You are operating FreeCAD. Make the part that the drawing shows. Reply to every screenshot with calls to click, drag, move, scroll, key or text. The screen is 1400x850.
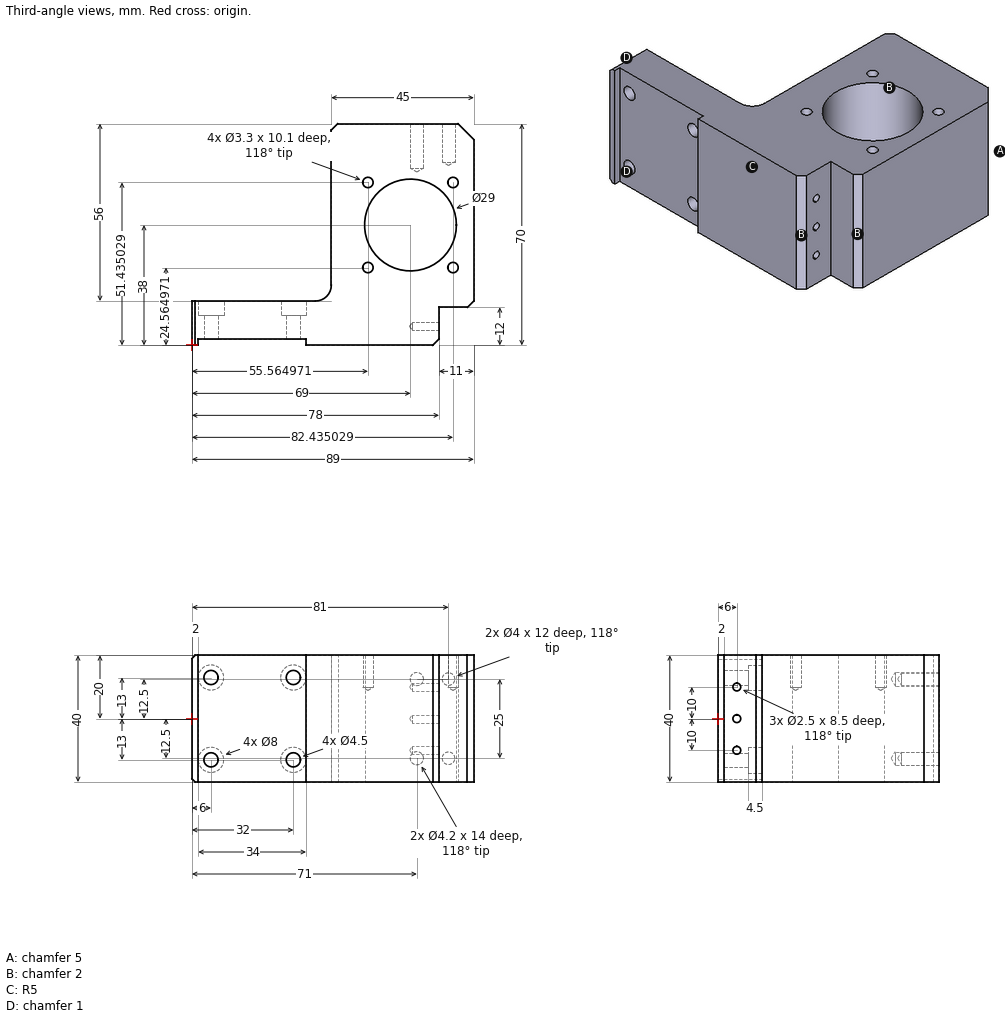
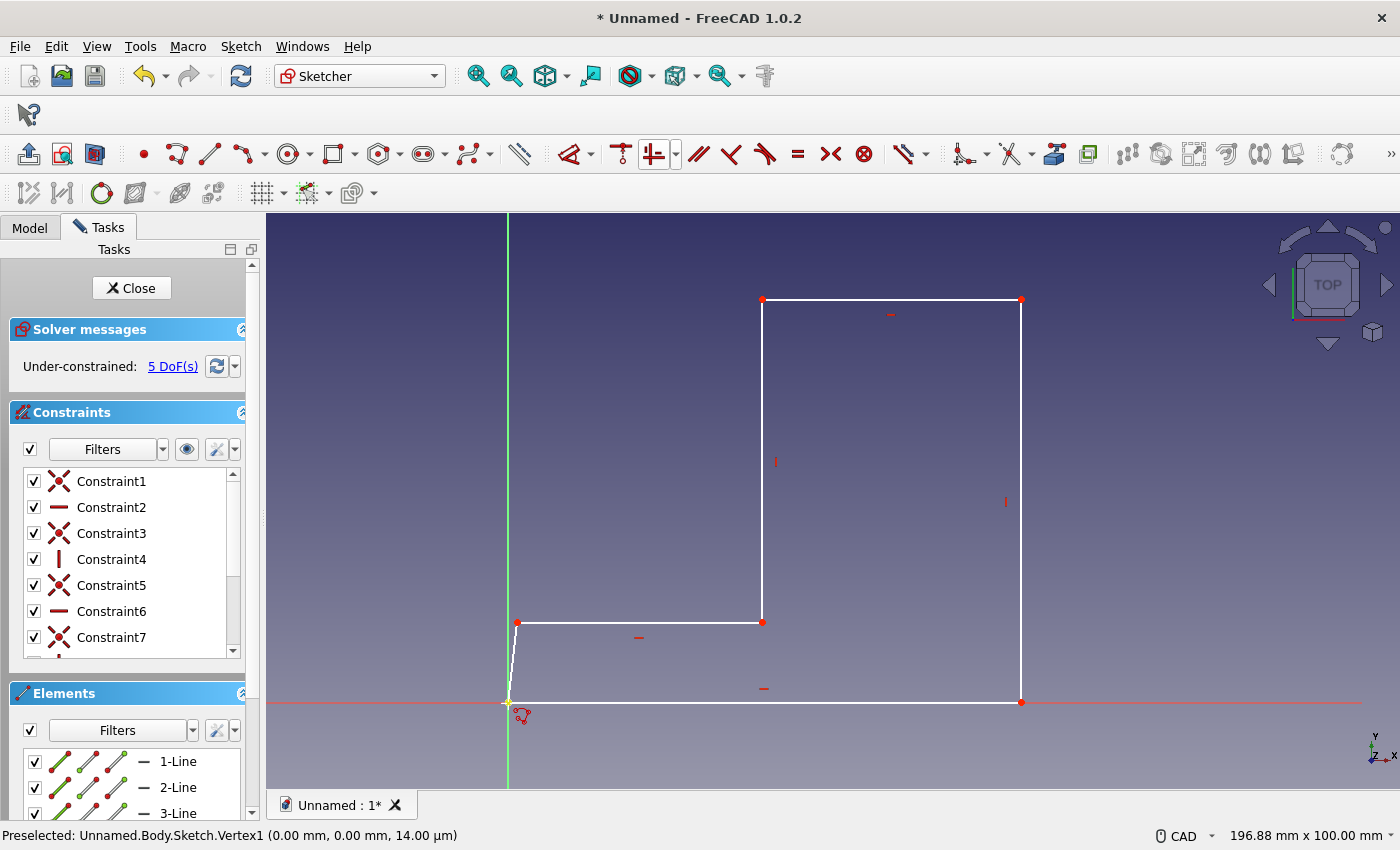
click(288, 154)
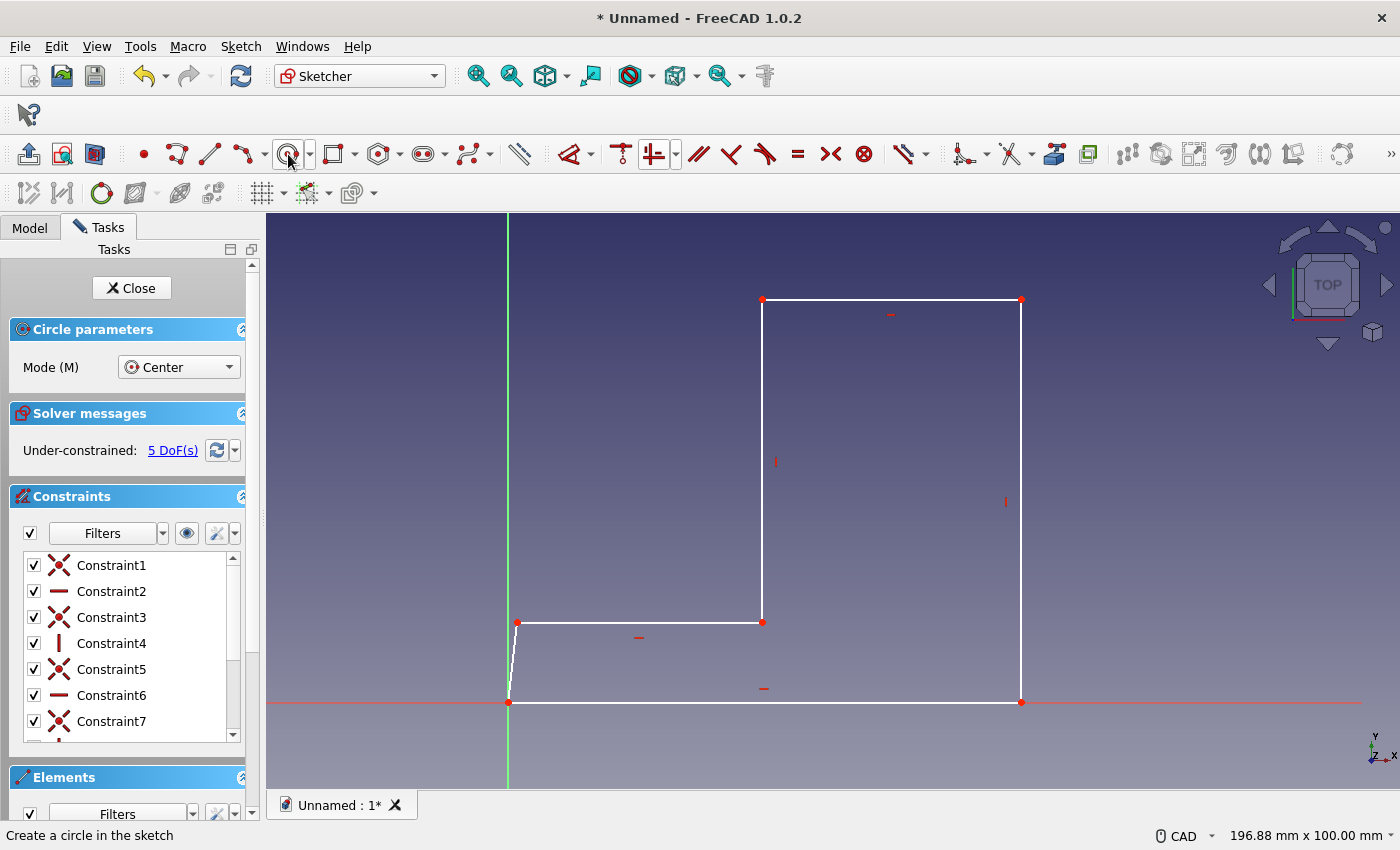
click(906, 484)
move(965, 425)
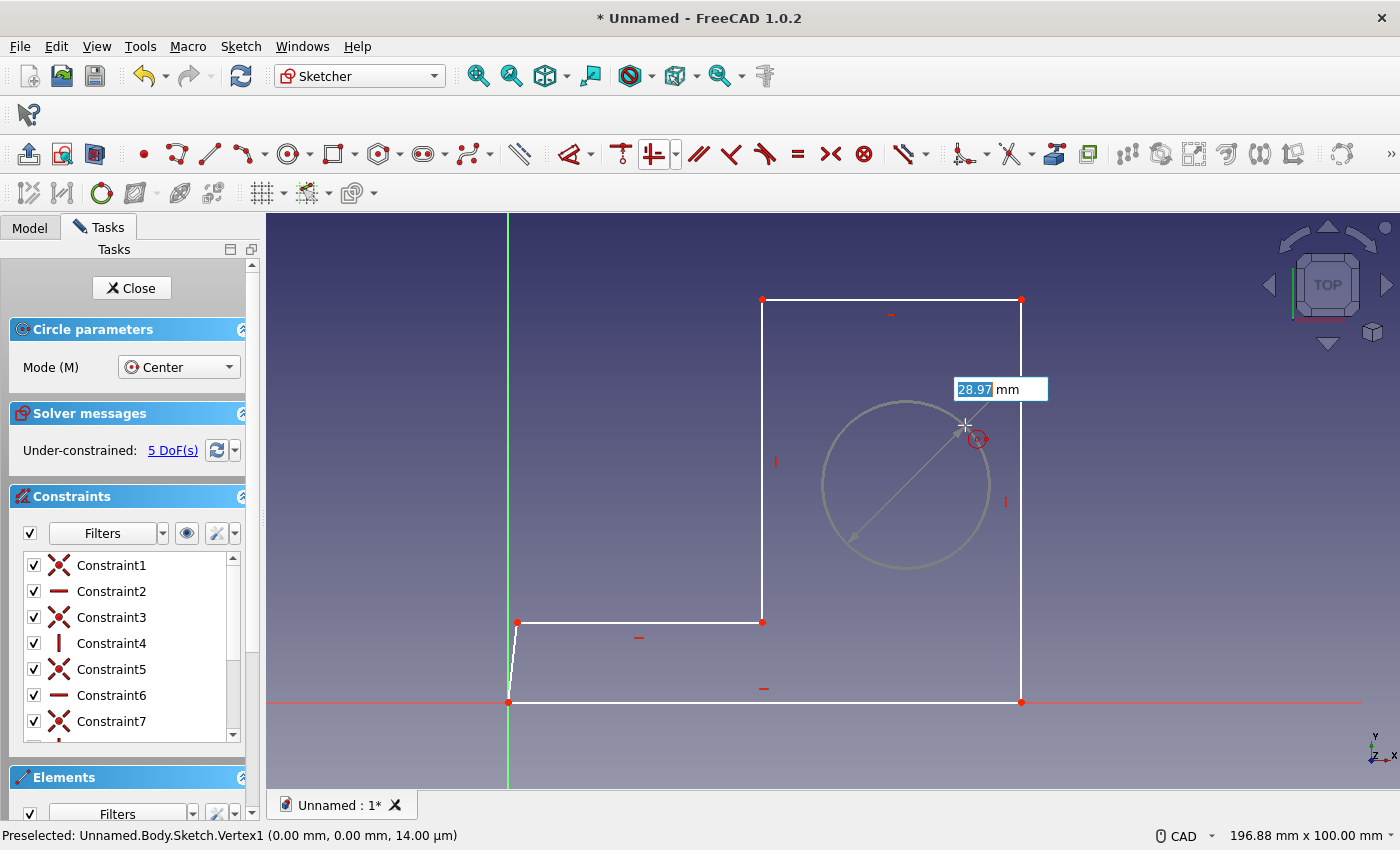
text(29)
key(Return)
key(Escape)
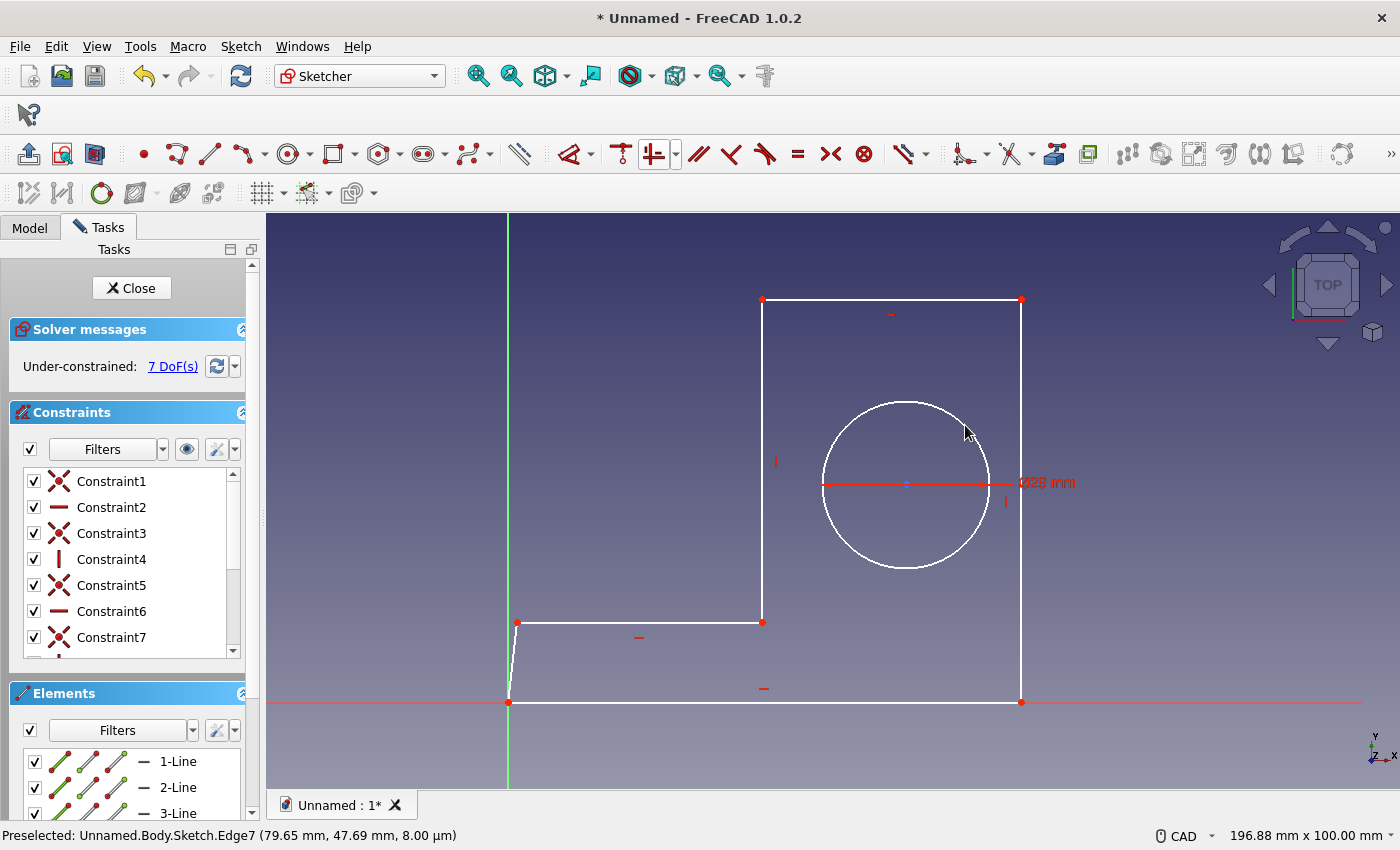
click(511, 679)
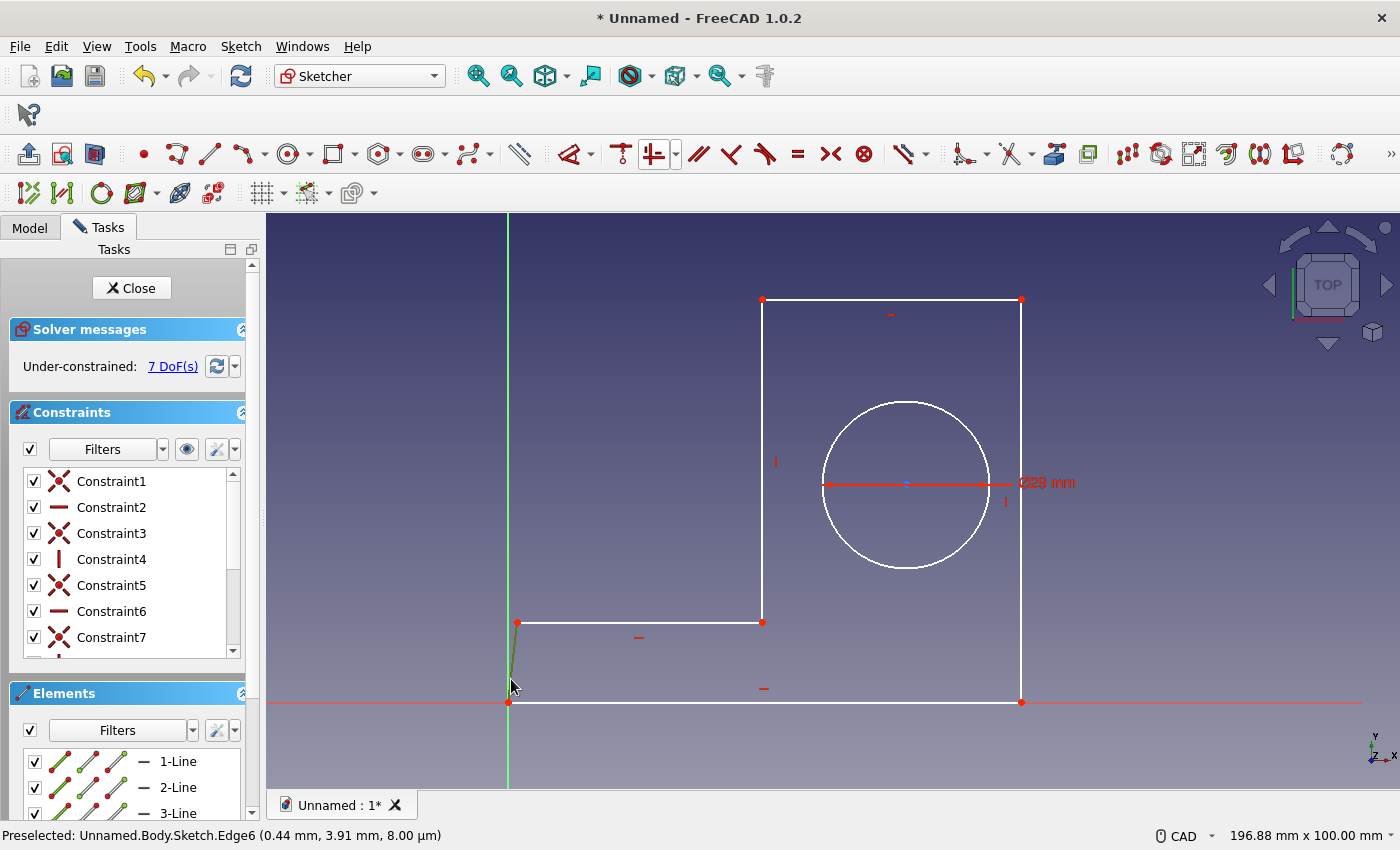
click(676, 154)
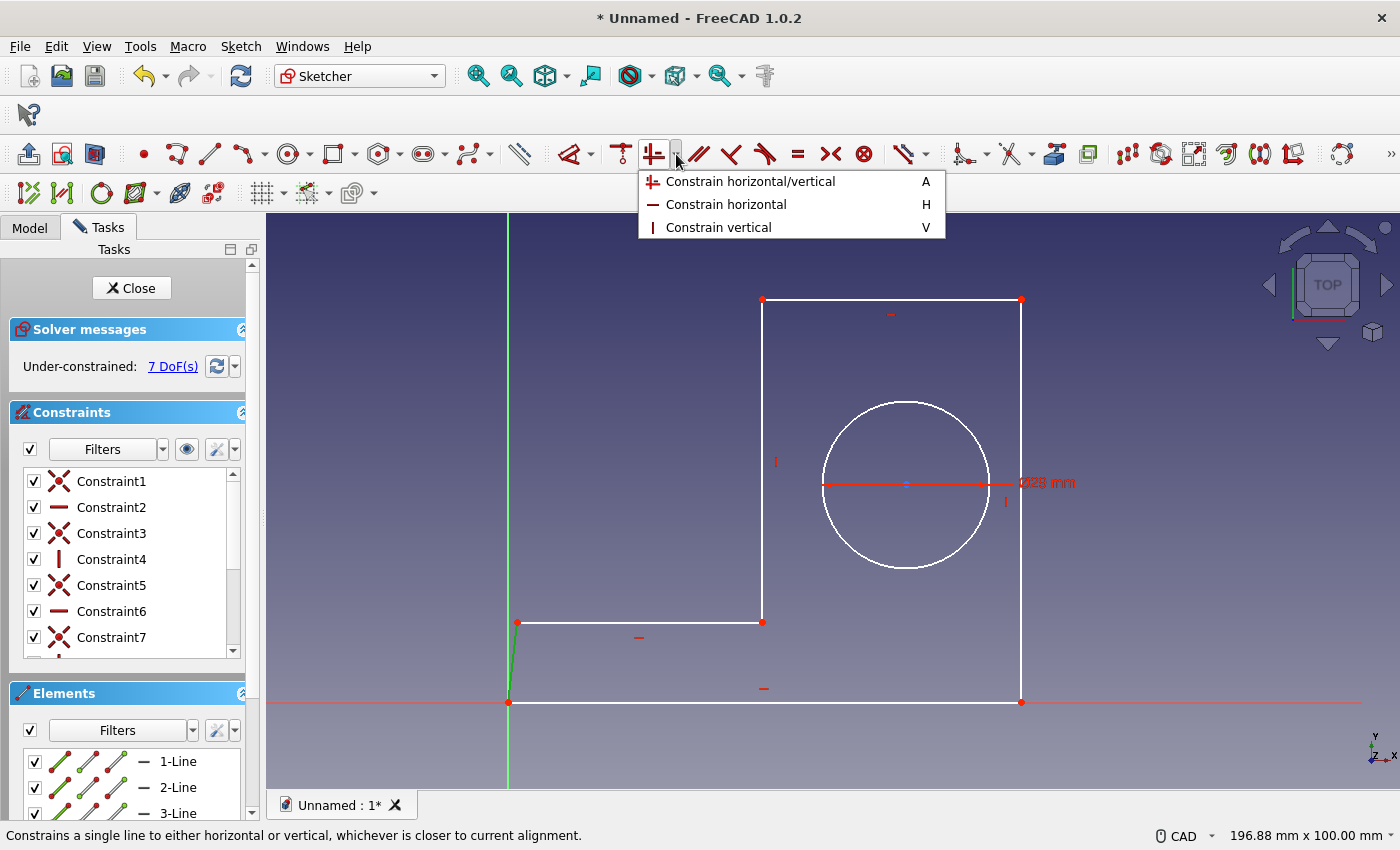
click(792, 228)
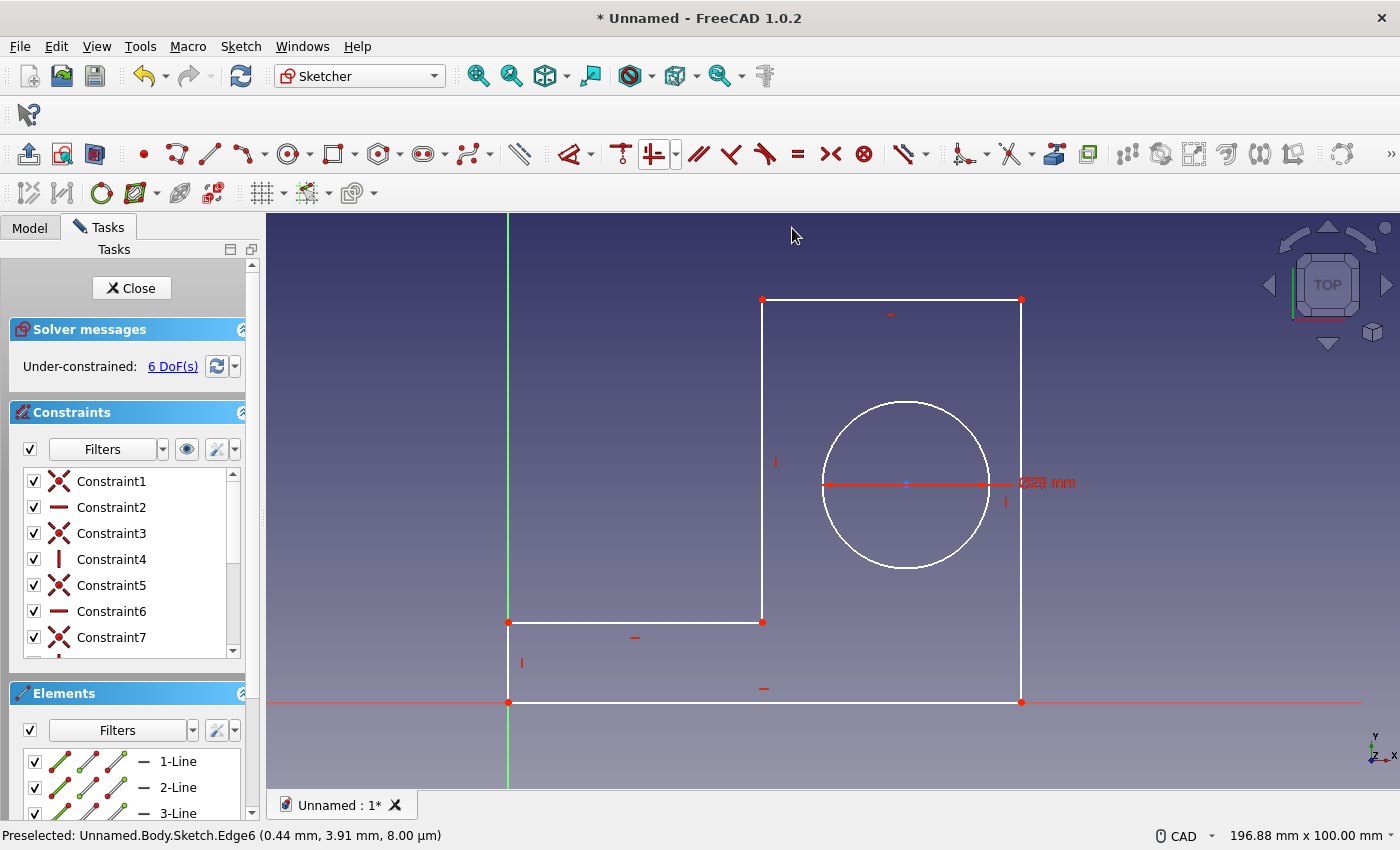
key(d)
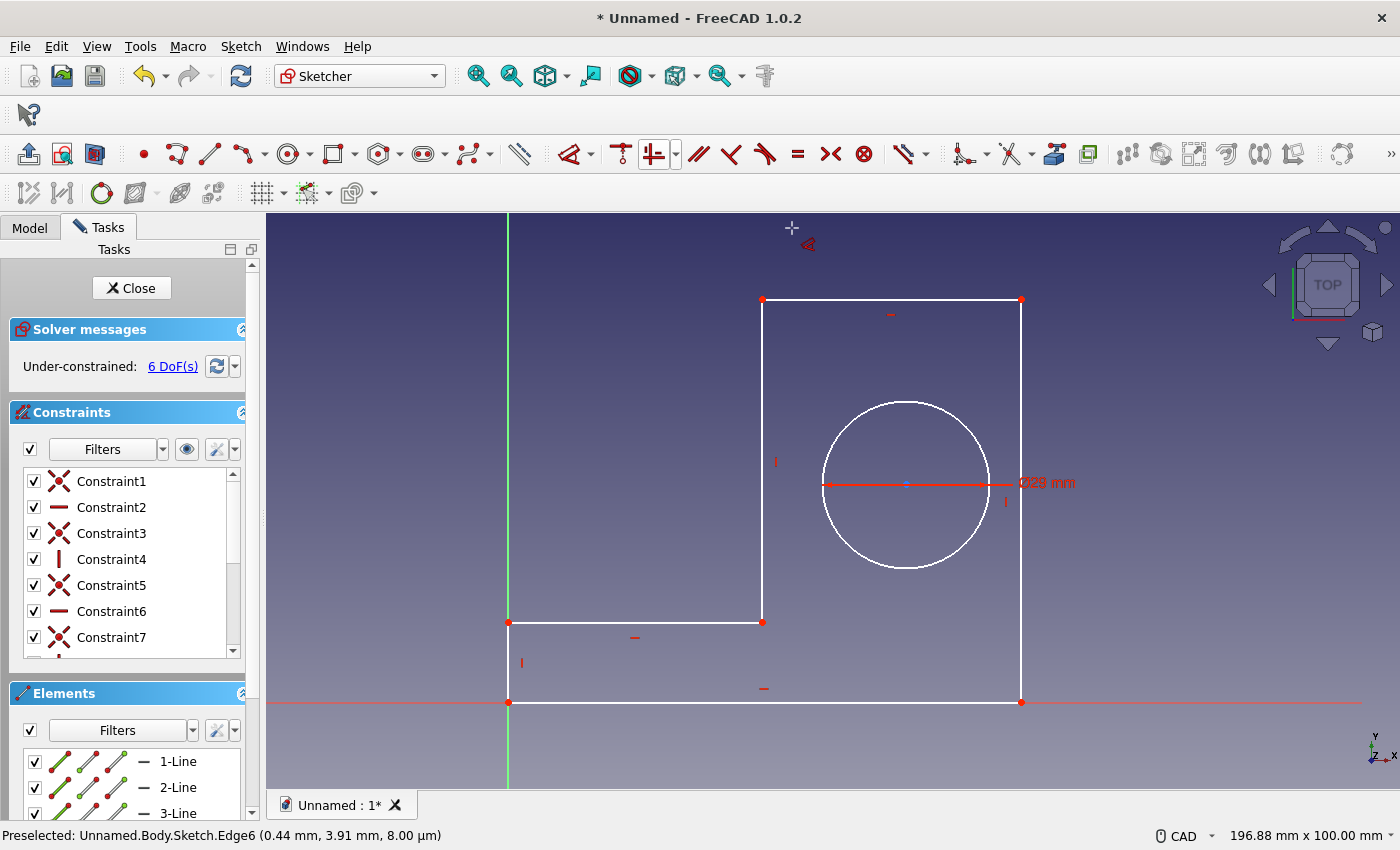
click(662, 703)
click(765, 737)